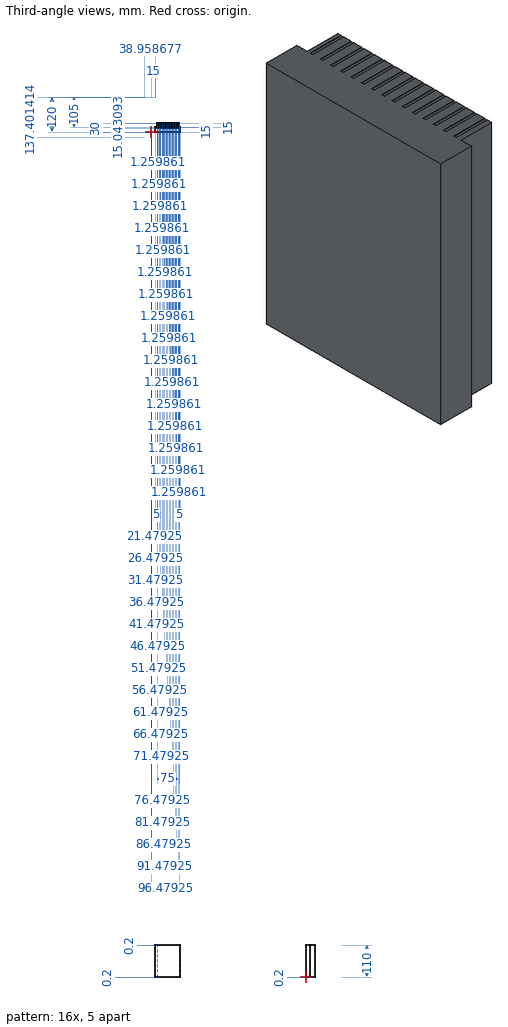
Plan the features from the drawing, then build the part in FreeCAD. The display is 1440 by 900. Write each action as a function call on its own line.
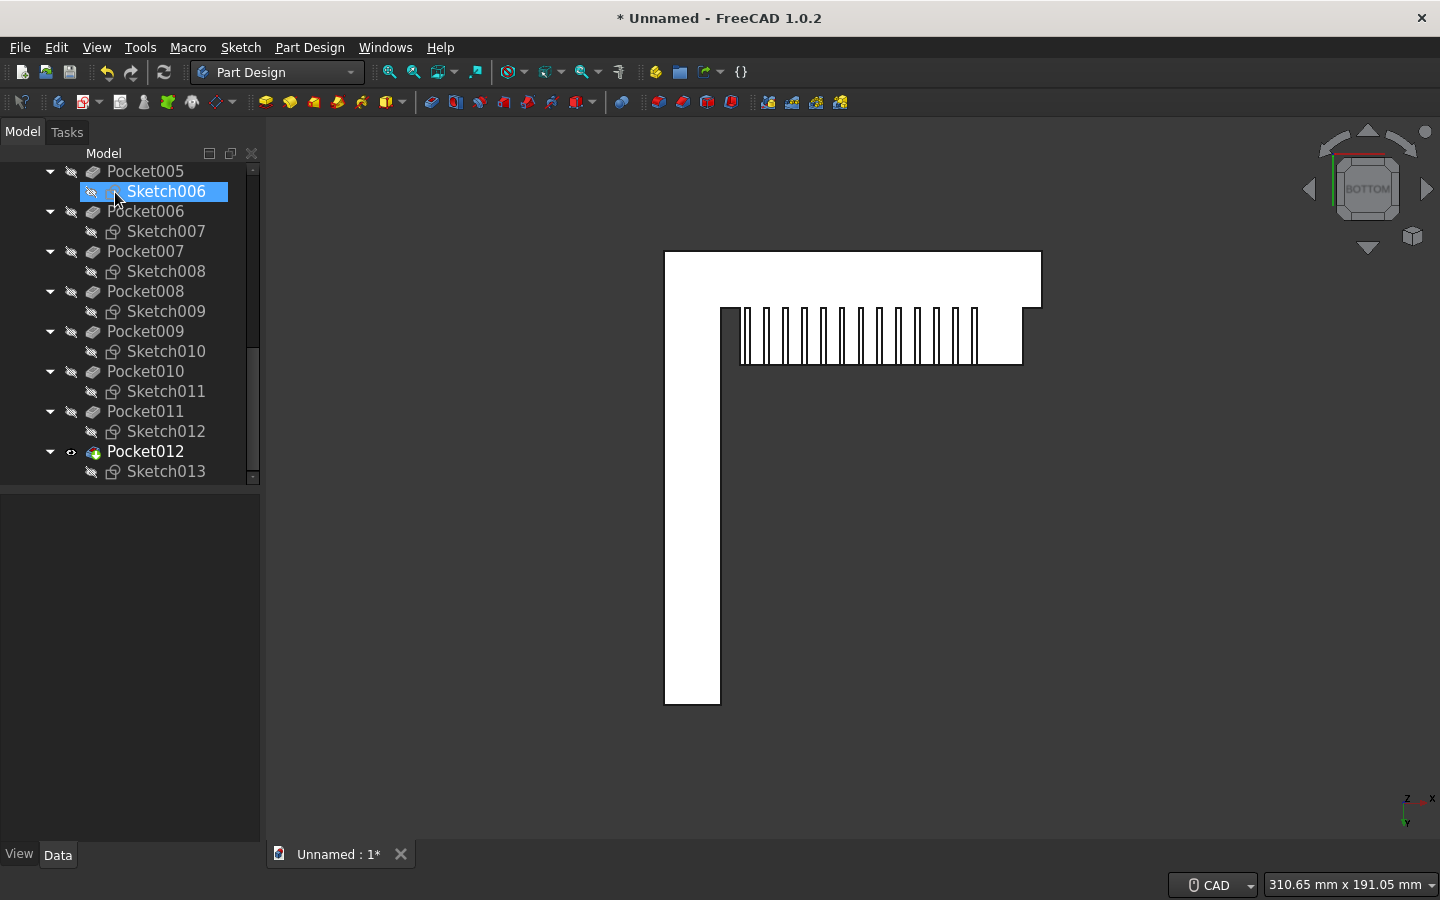
click(84, 102)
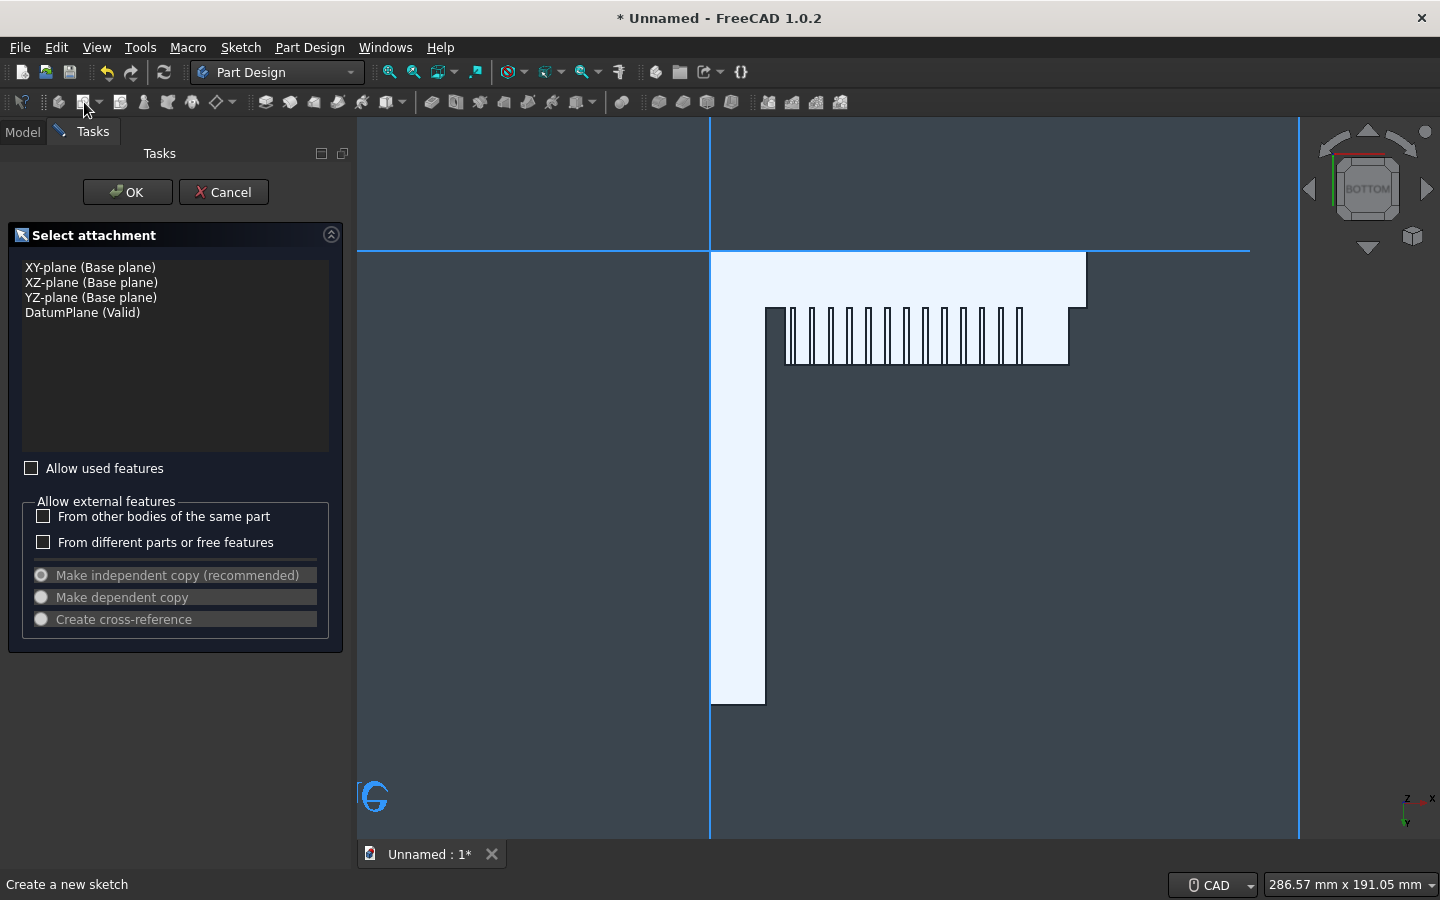
click(82, 268)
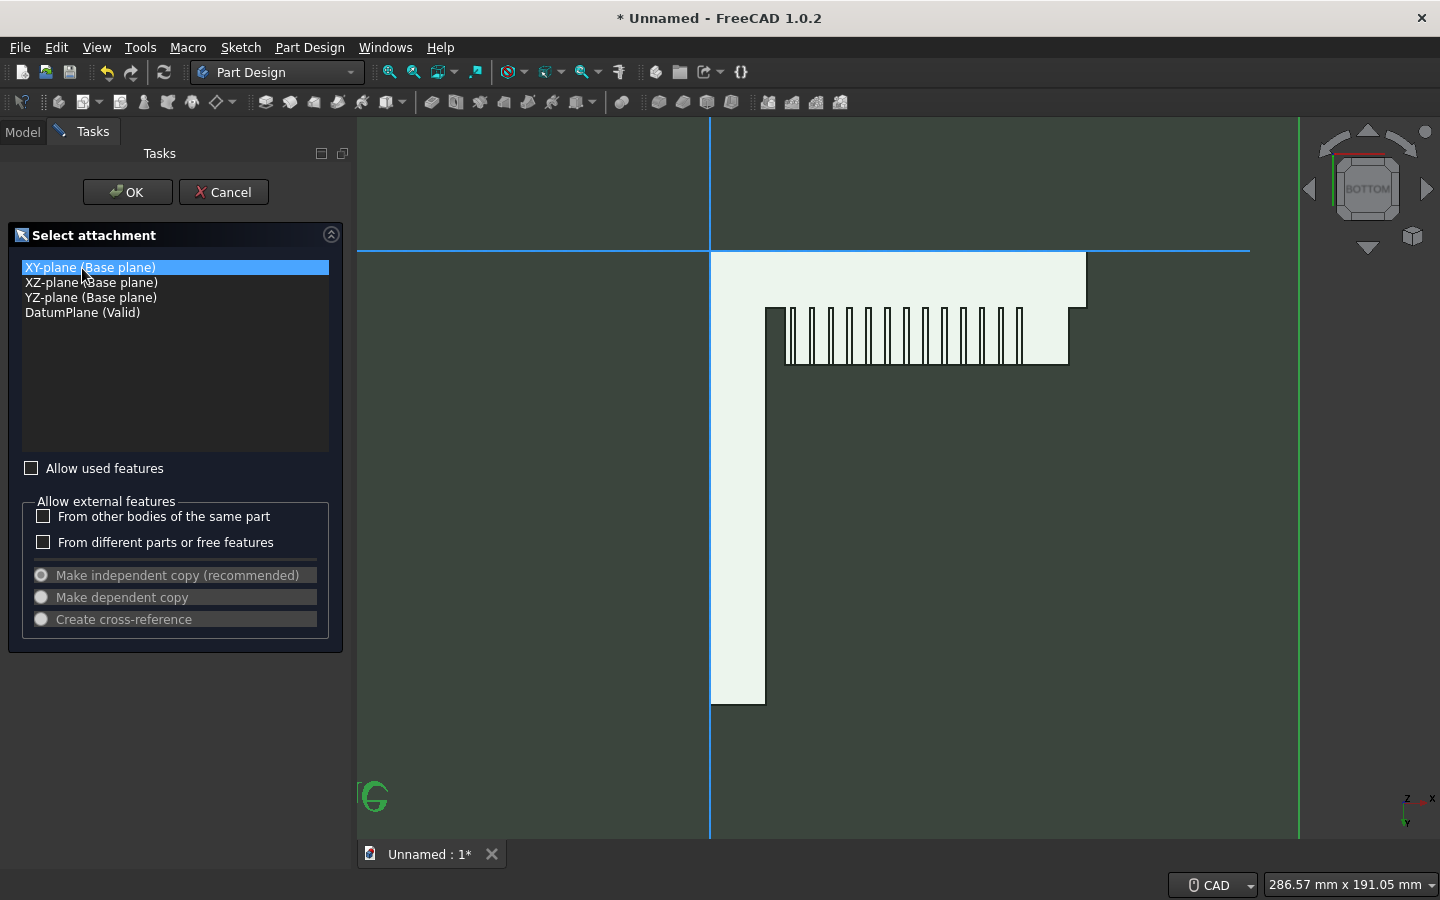
click(128, 192)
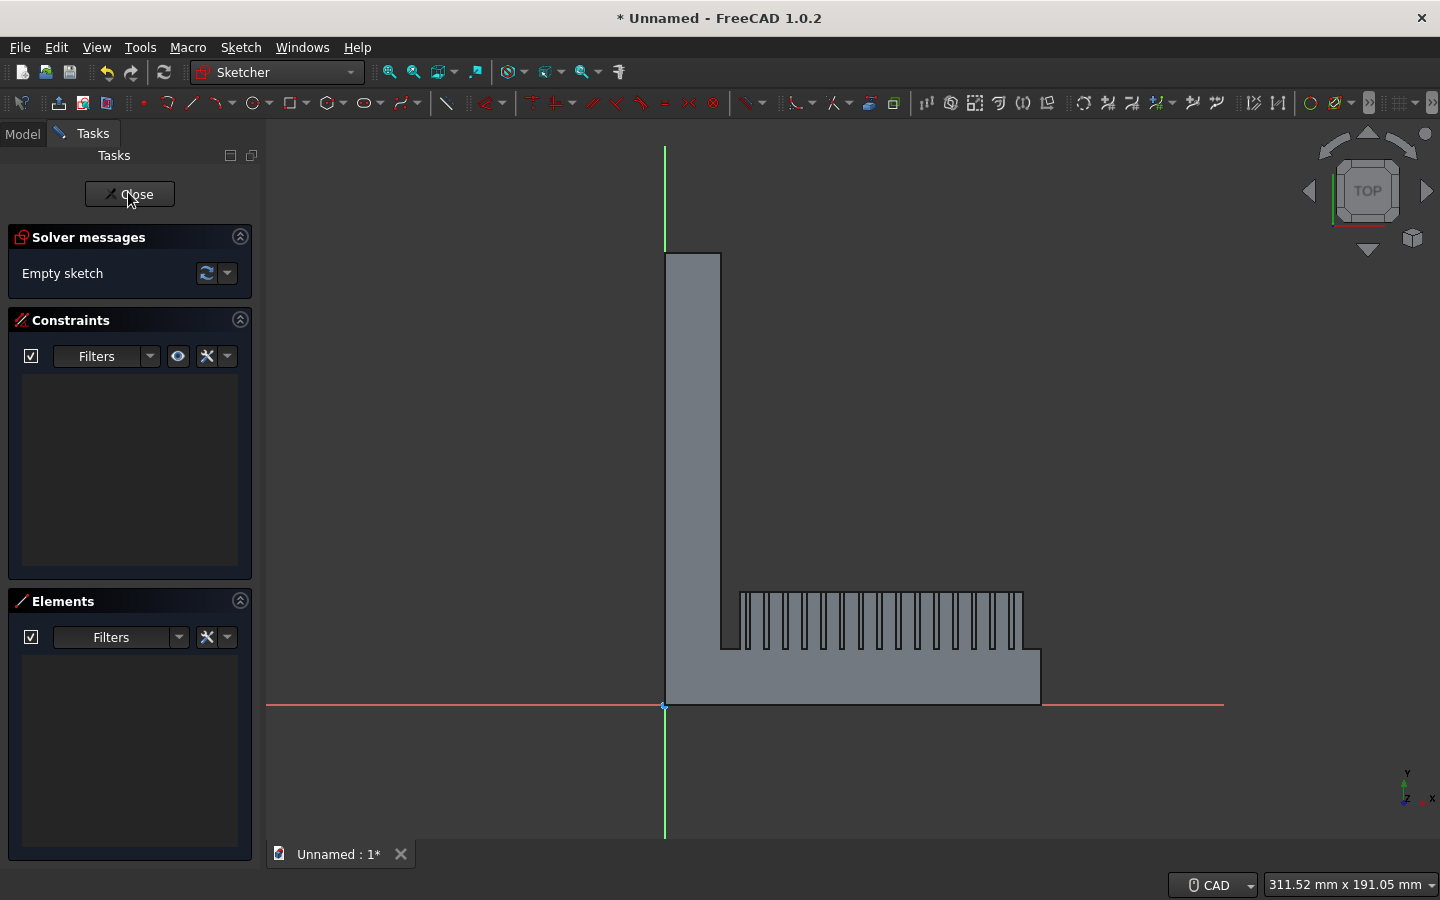
click(108, 104)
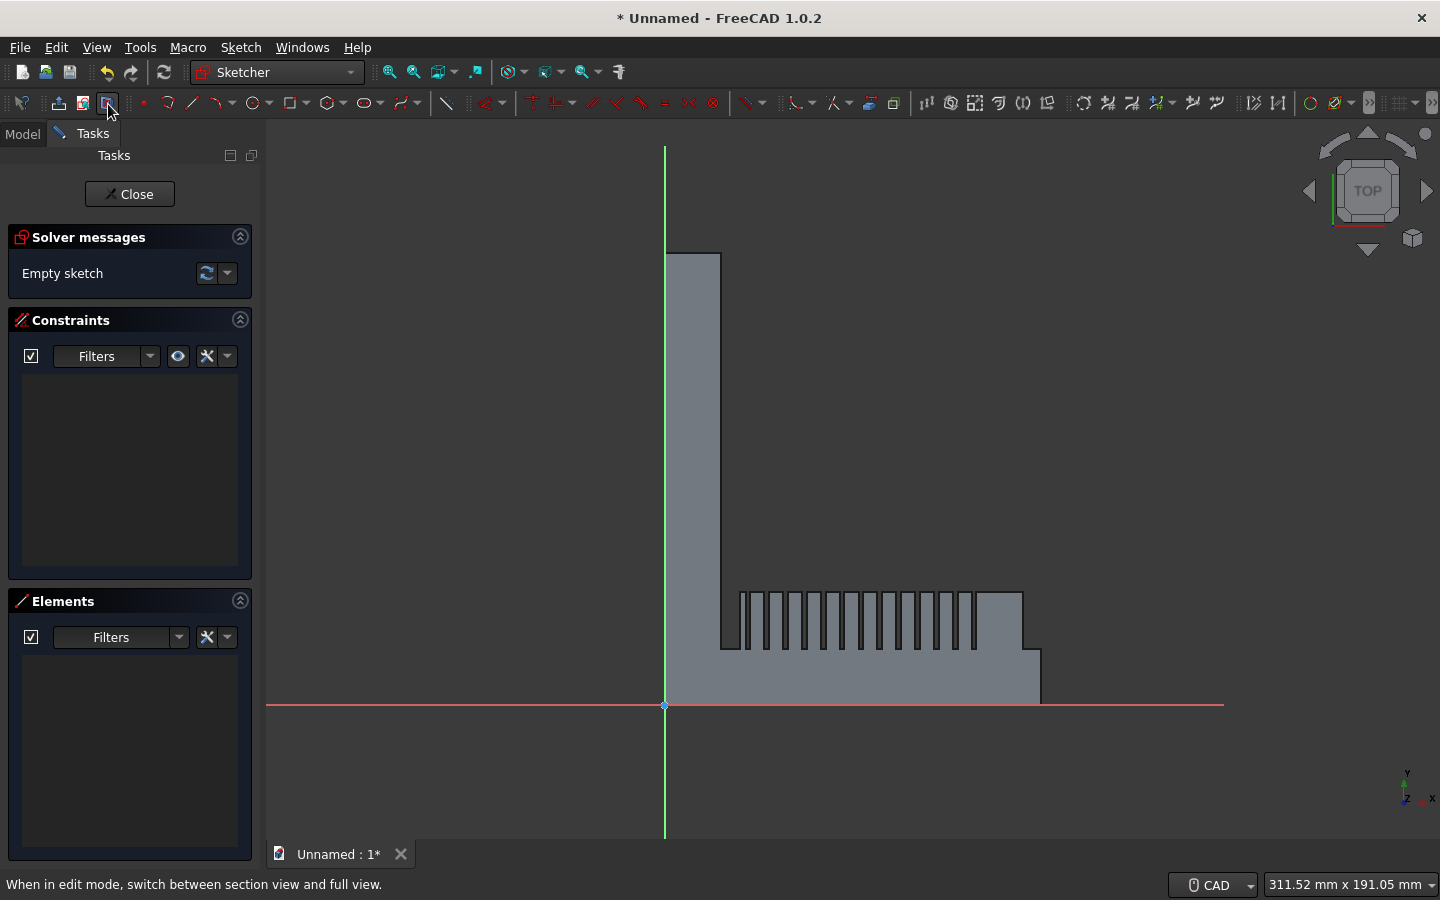
scroll(1019, 638, up, 11)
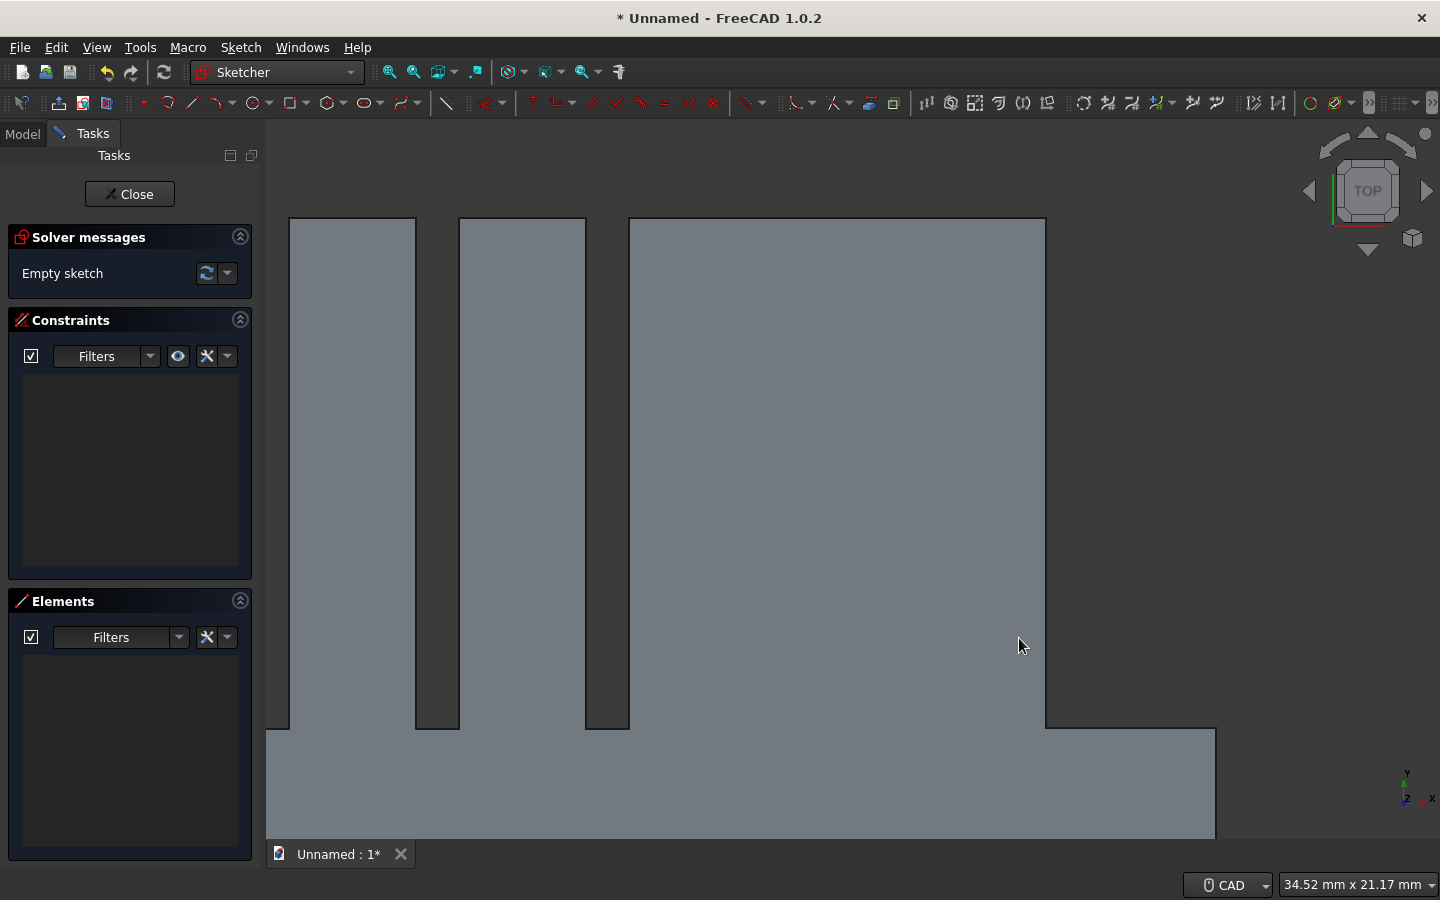
key(g)
key(r)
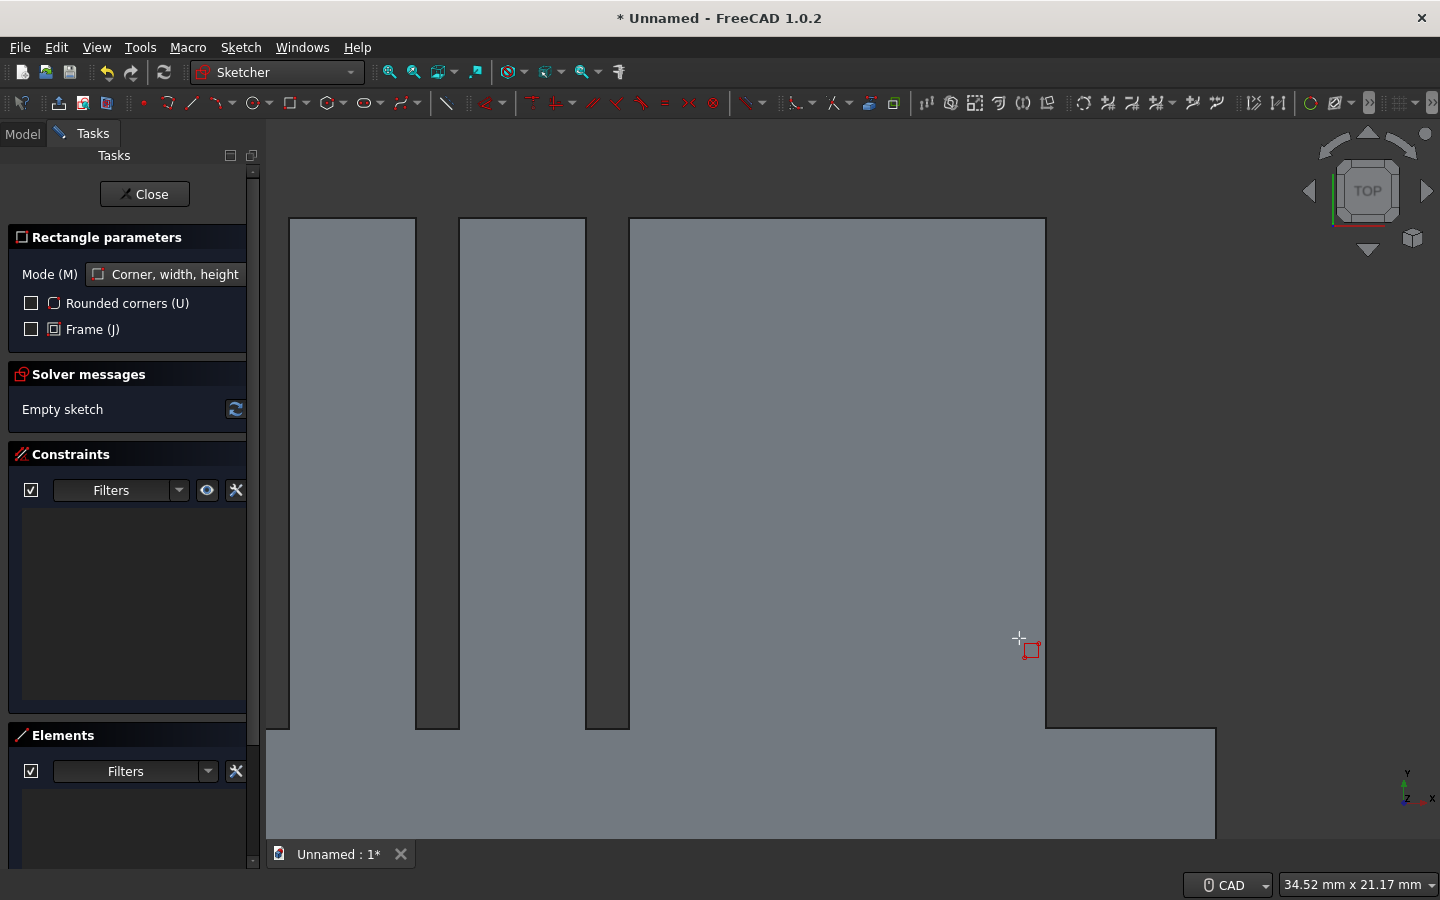
click(756, 218)
click(799, 729)
key(Escape)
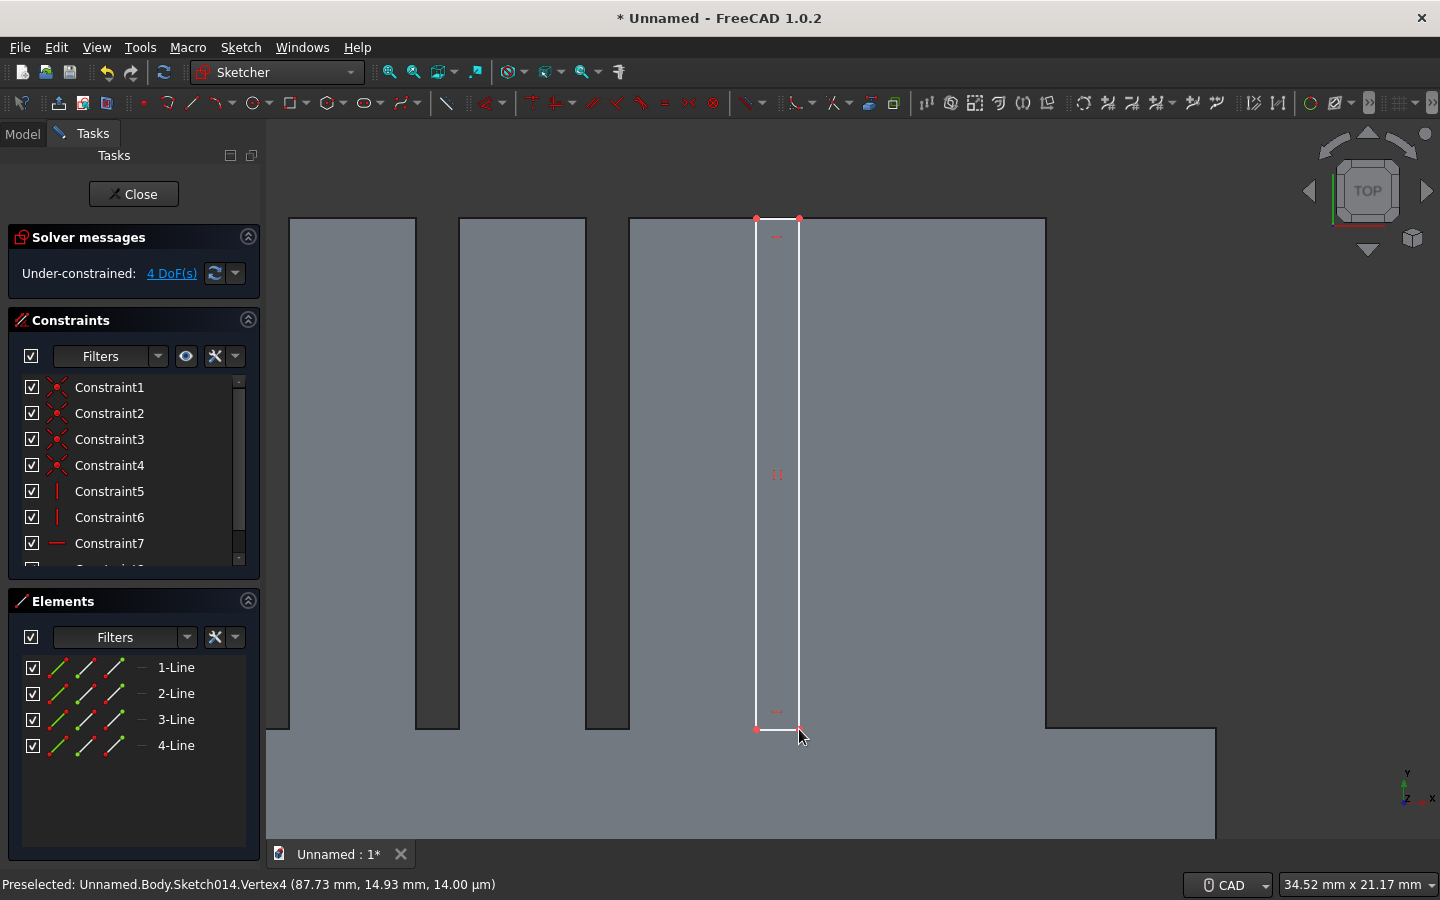
click(486, 104)